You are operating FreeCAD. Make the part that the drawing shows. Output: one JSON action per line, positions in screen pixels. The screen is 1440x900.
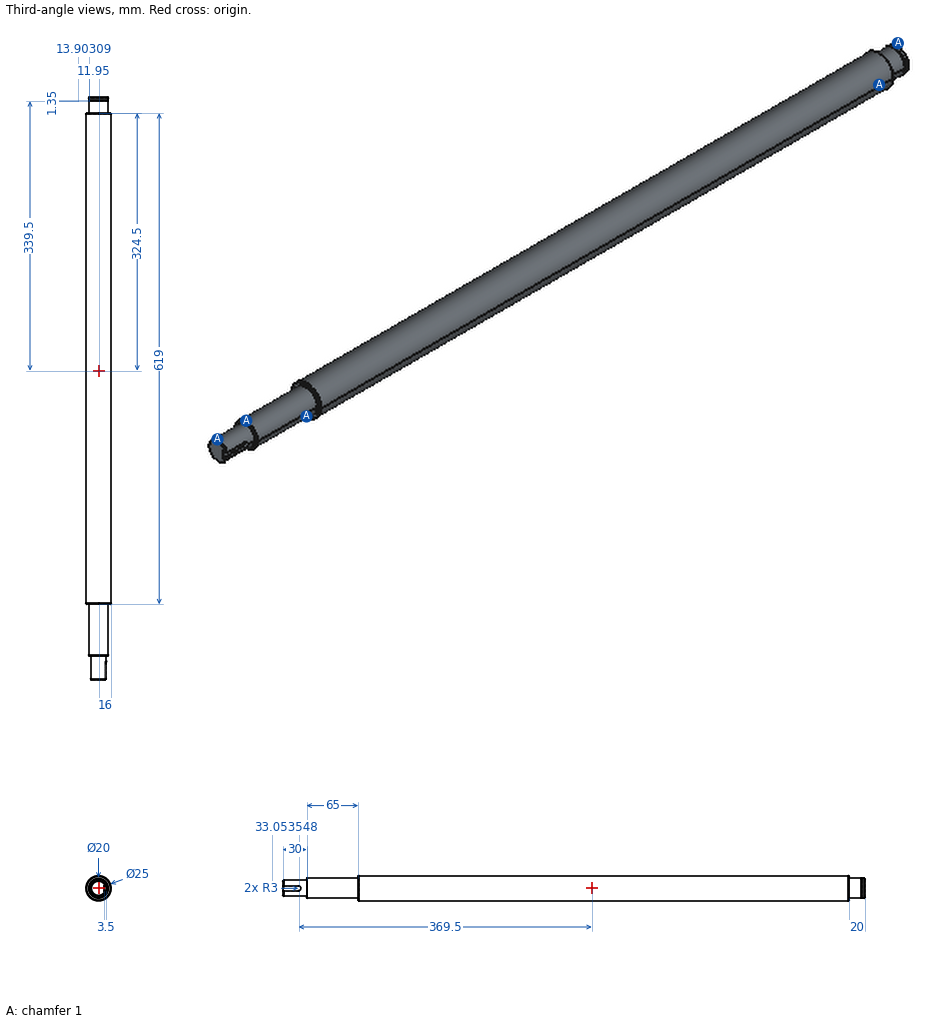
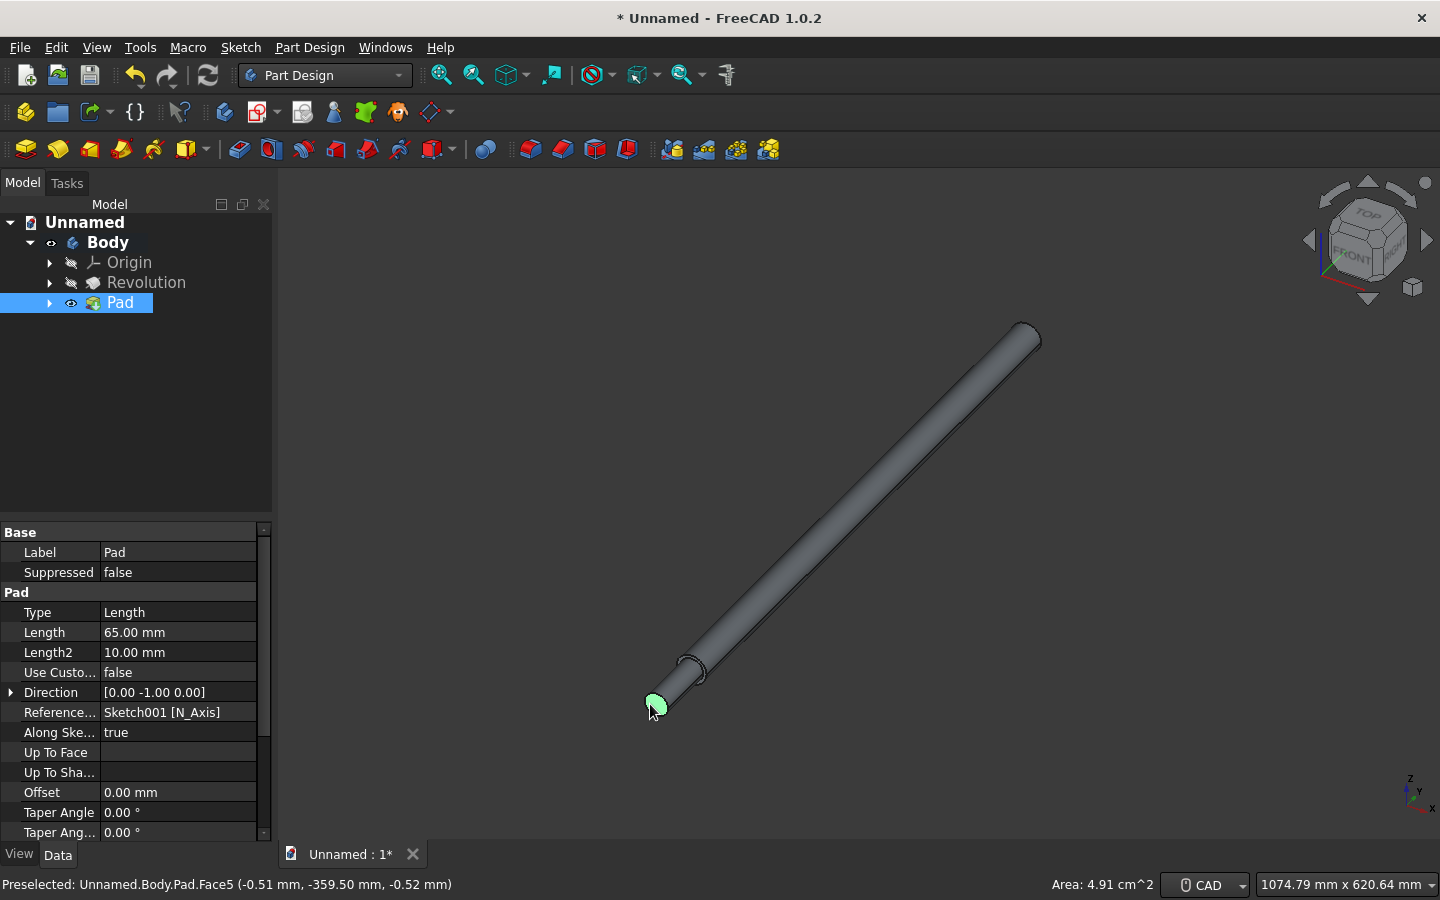
{"action": "left_click", "coordinate": [258, 112]}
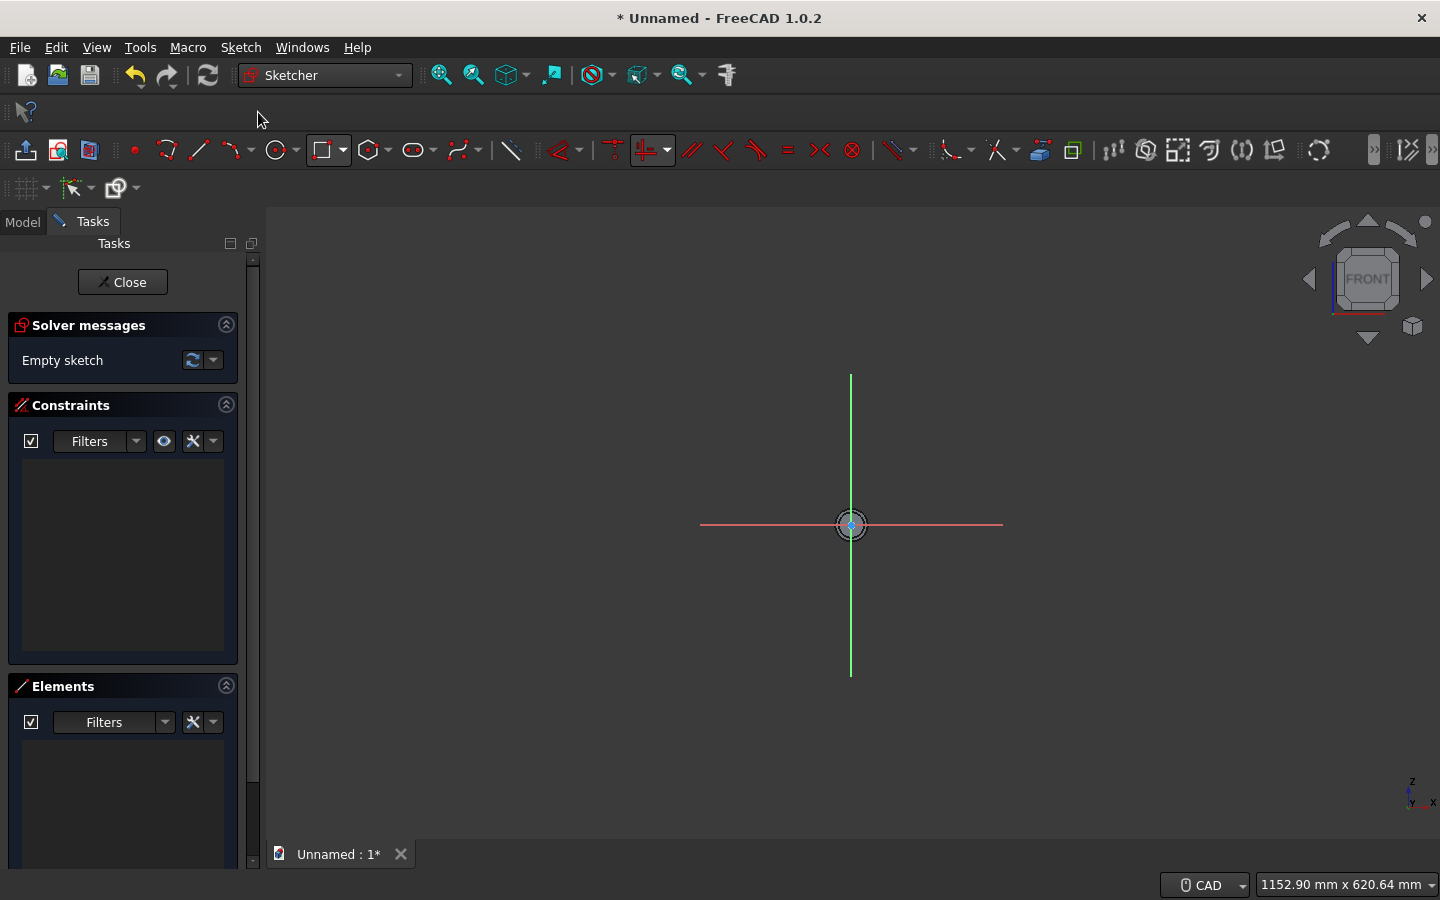
{"action": "scroll", "coordinate": [855, 525], "scroll_direction": "up", "scroll_amount": 15}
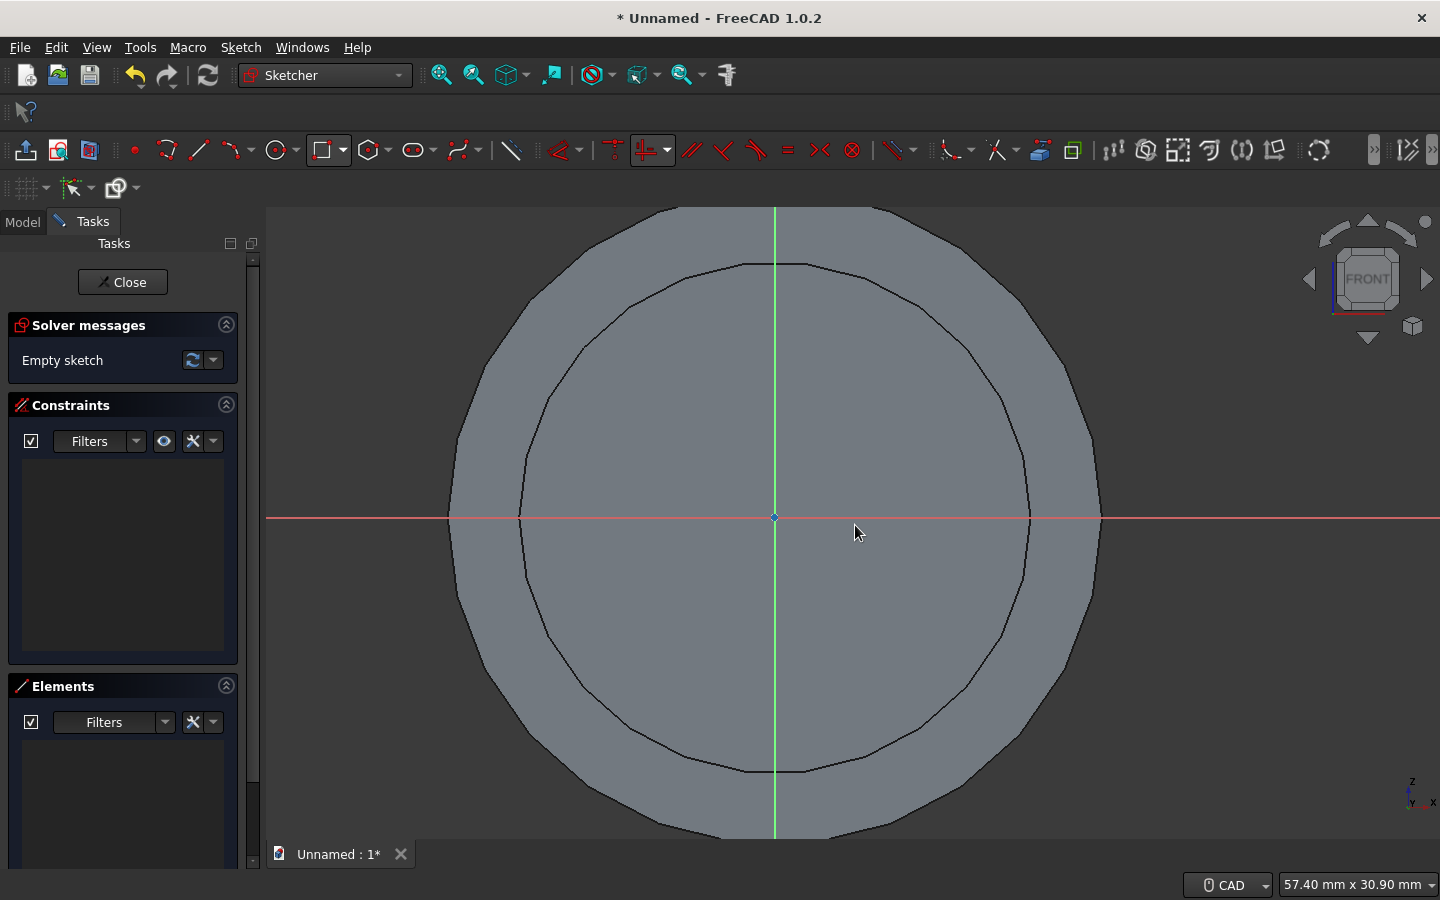
{"action": "left_click", "coordinate": [276, 150]}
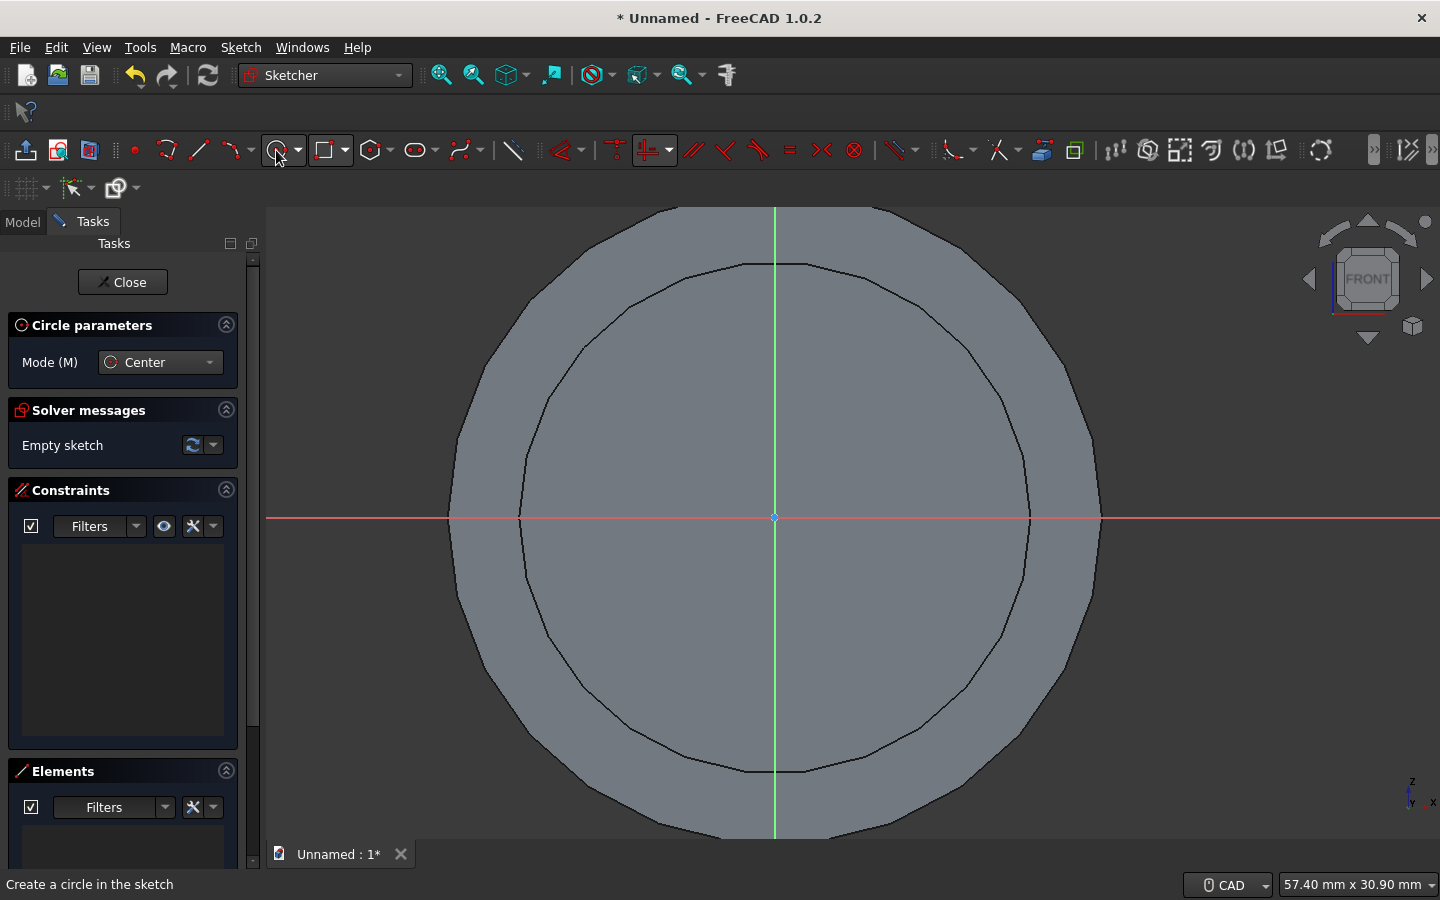
{"action": "left_click", "coordinate": [775, 518]}
{"action": "mouse_move", "coordinate": [920, 373]}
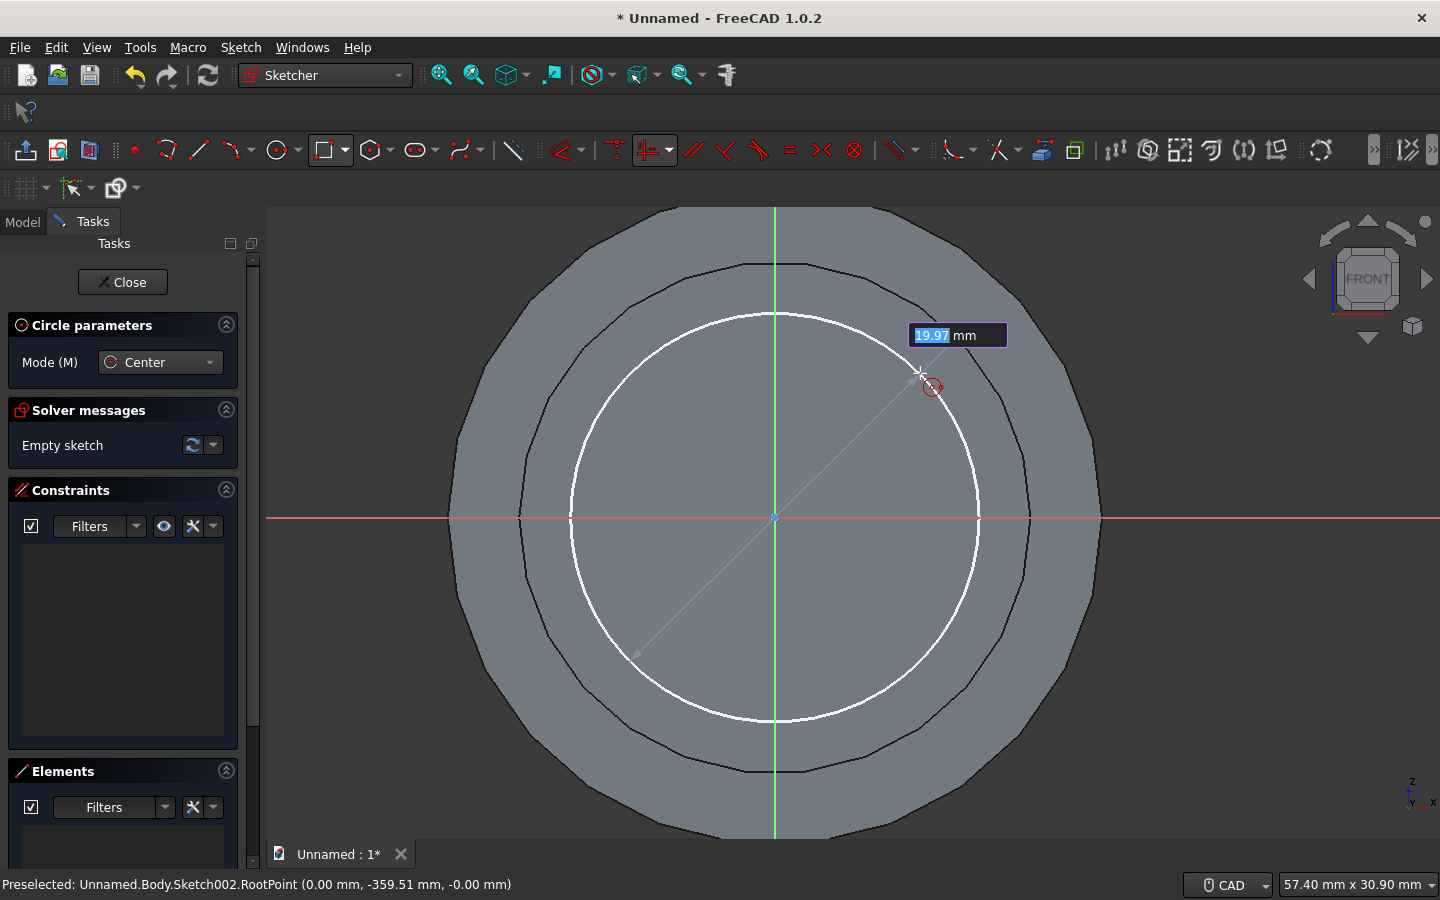
{"action": "type", "text": "20"}
{"action": "key", "text": "Return"}
{"action": "key", "text": "Escape"}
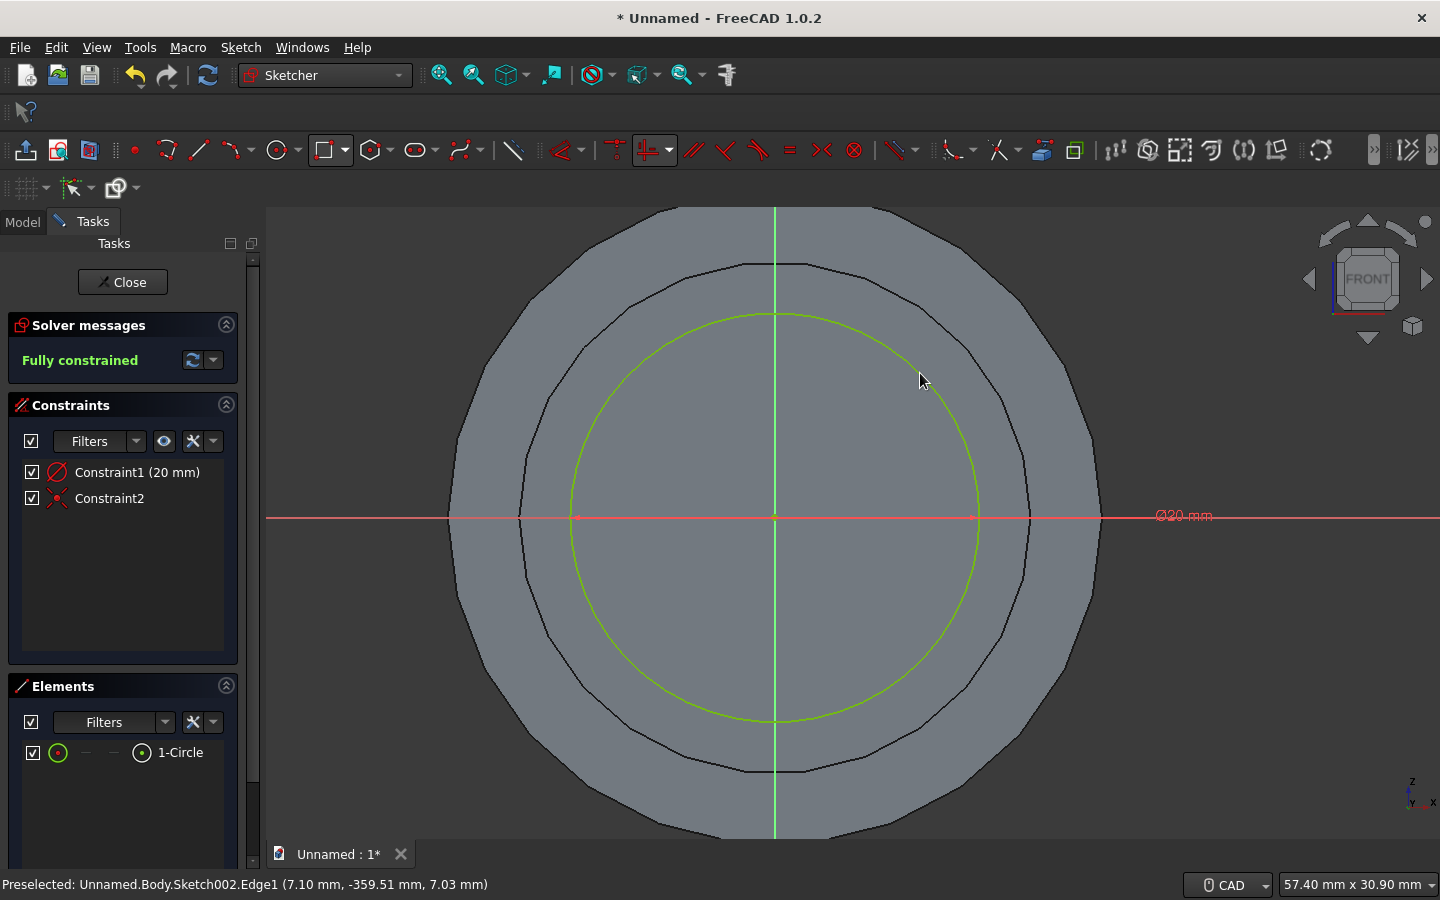
{"action": "left_click", "coordinate": [123, 282]}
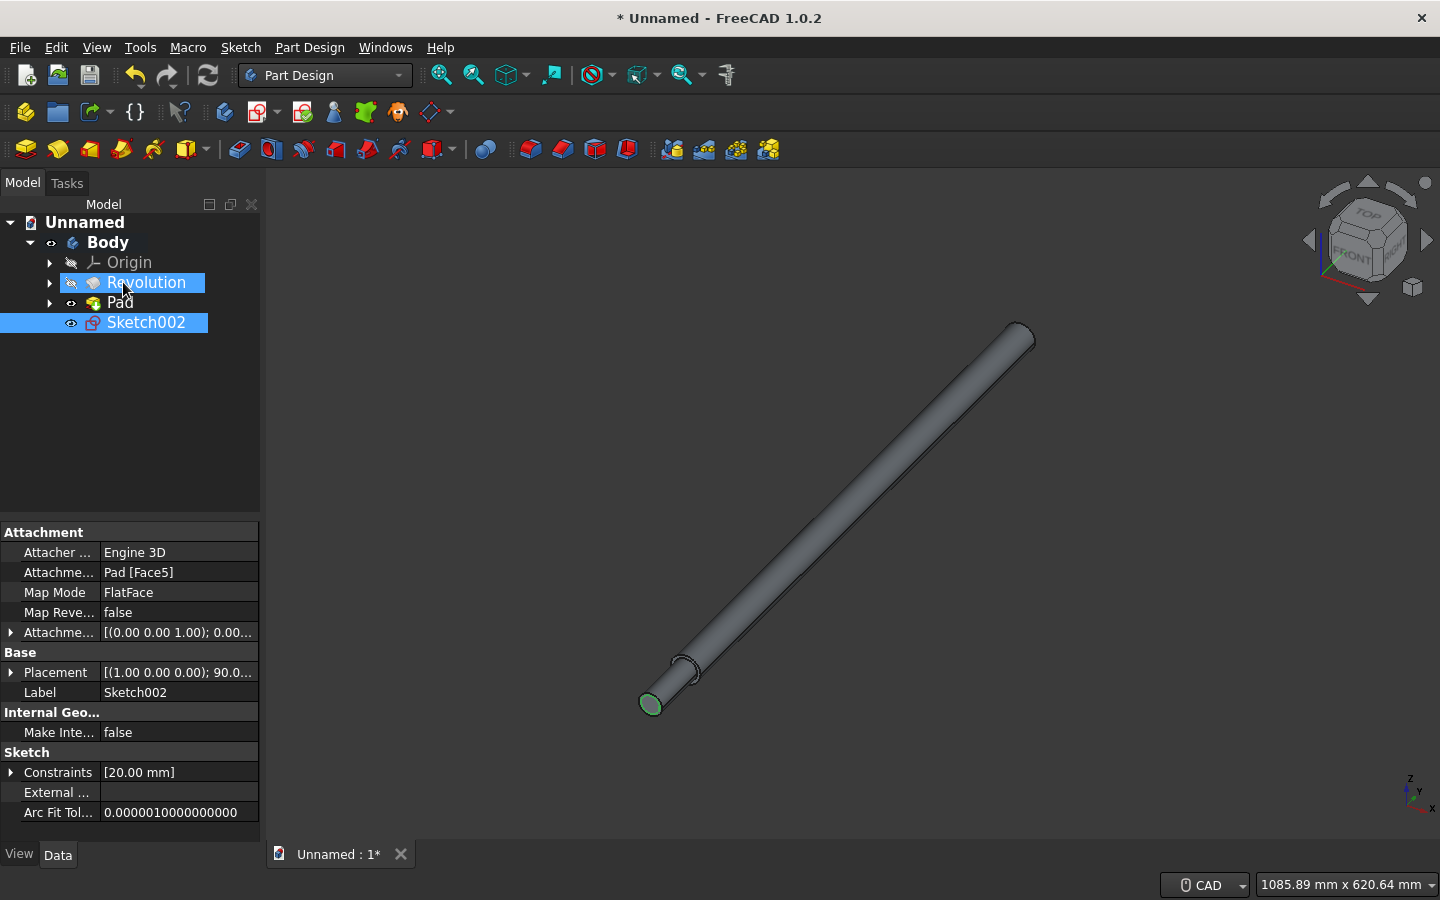
{"action": "left_click", "coordinate": [26, 150]}